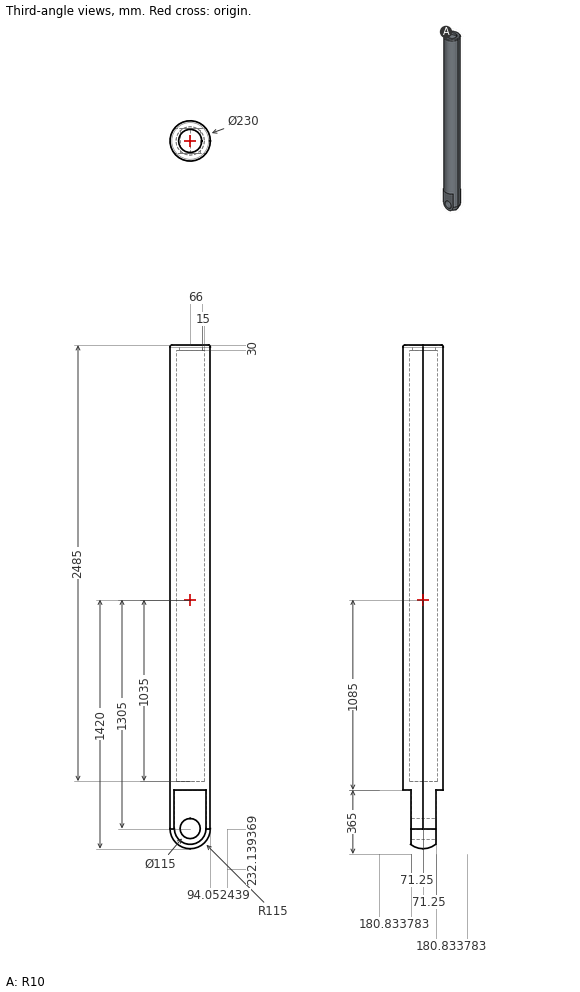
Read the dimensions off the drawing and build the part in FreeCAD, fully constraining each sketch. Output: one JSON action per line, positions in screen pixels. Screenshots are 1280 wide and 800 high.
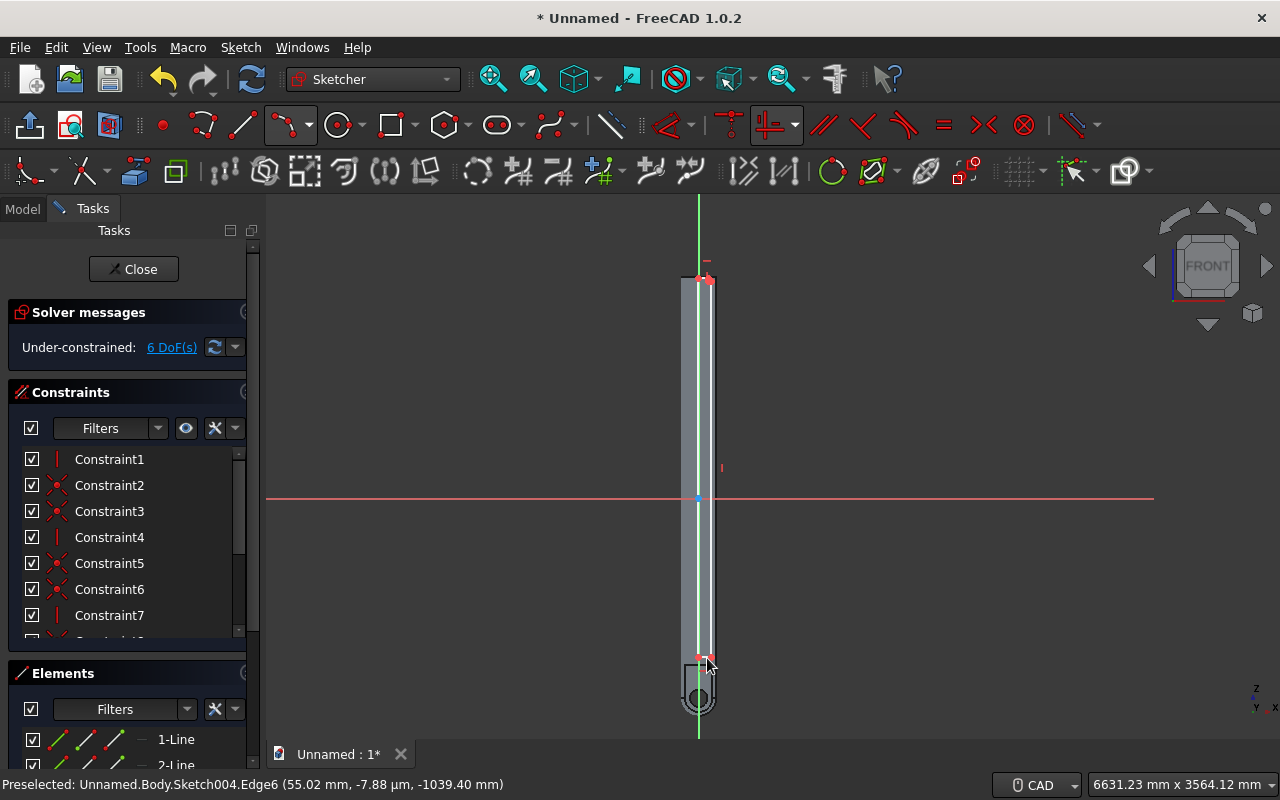
{"action": "left_click", "coordinate": [698, 657]}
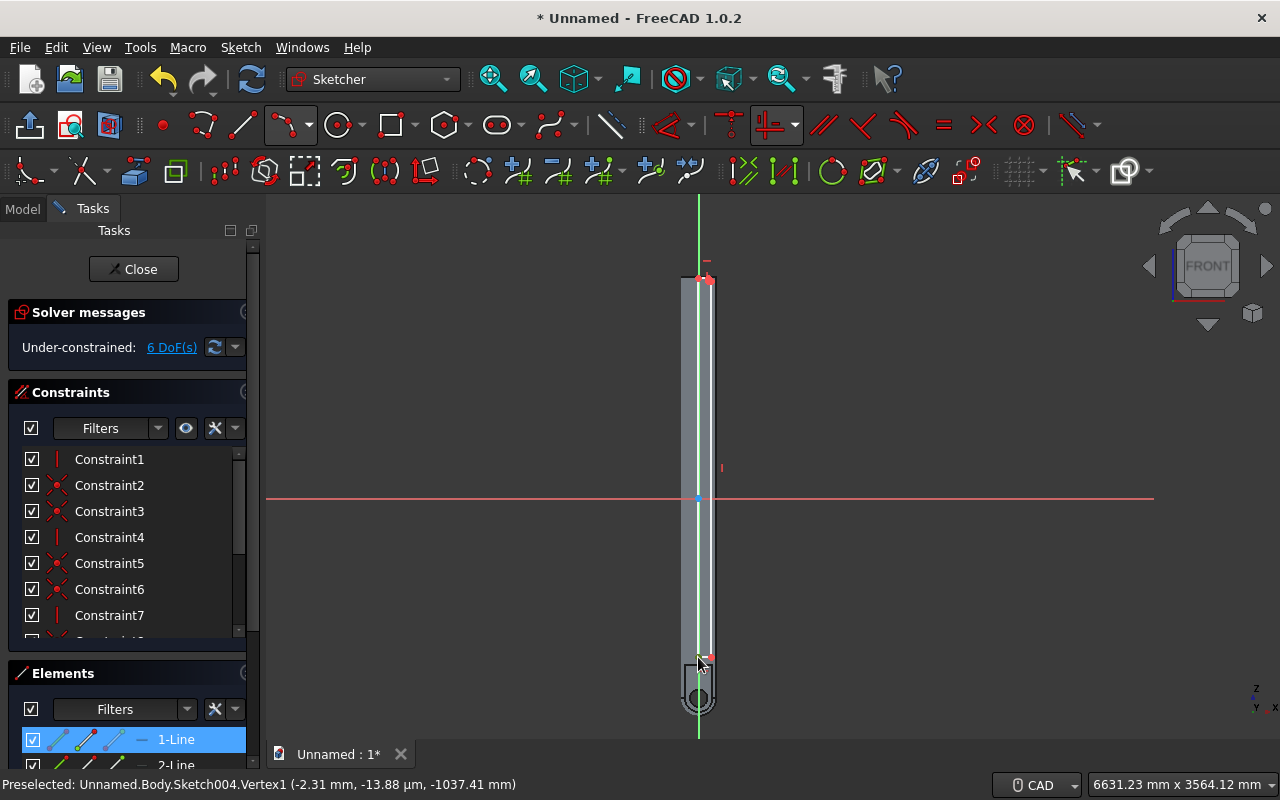
{"action": "left_click", "coordinate": [699, 257]}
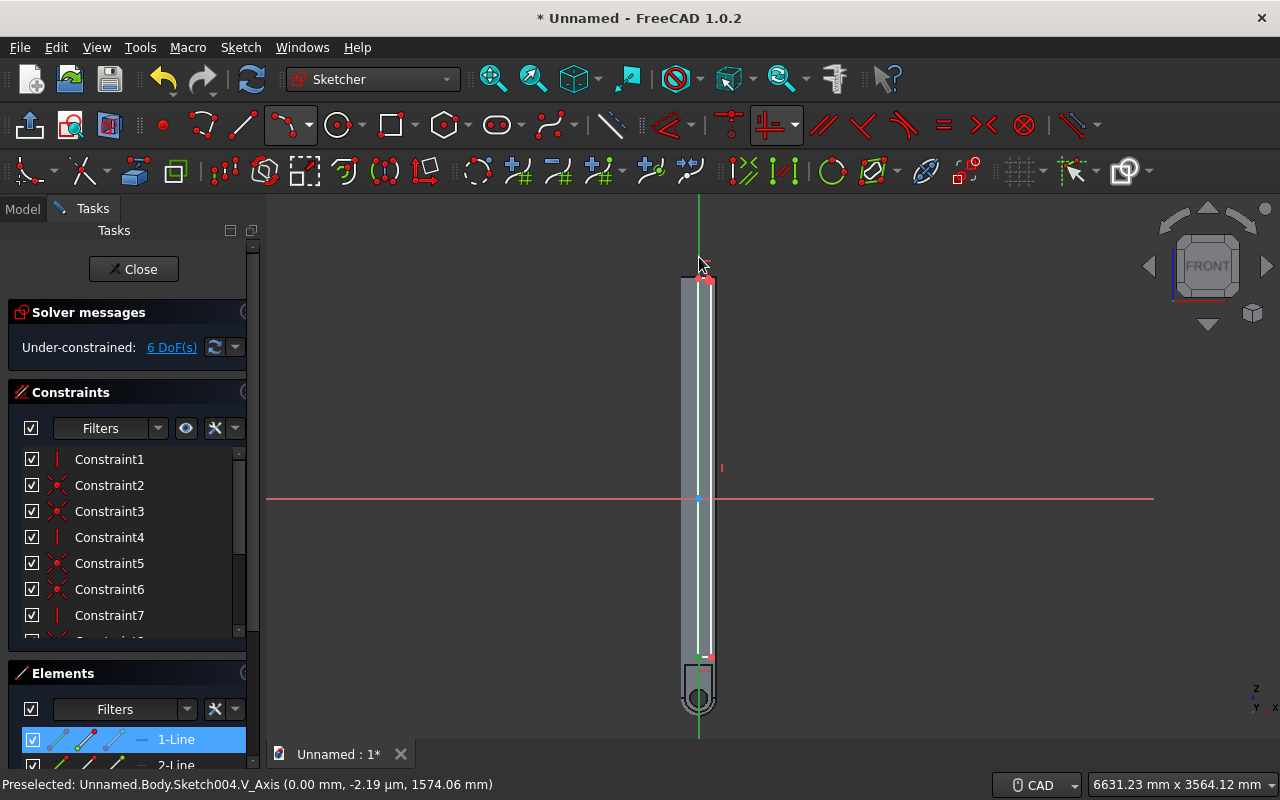
{"action": "key", "text": "c"}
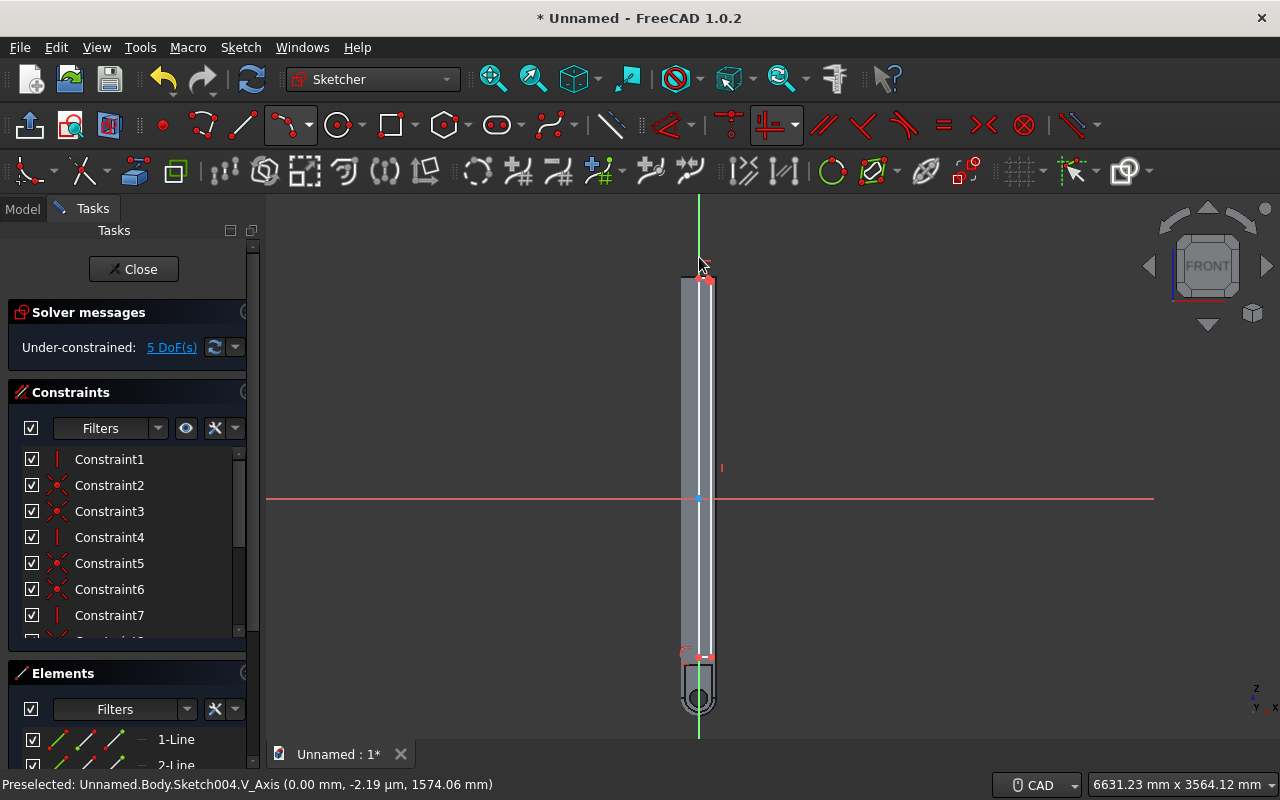
{"action": "key", "text": "d"}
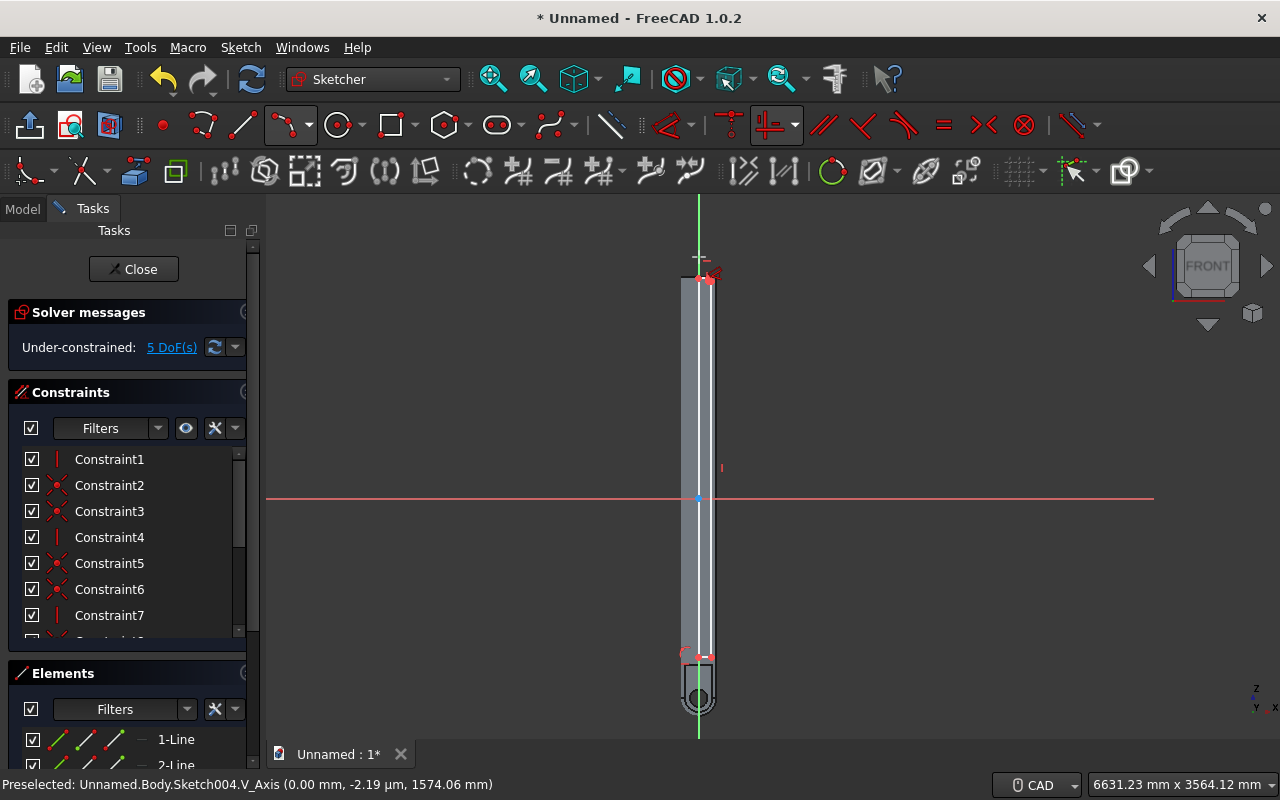
{"action": "scroll", "coordinate": [704, 278], "scroll_direction": "up", "scroll_amount": 7}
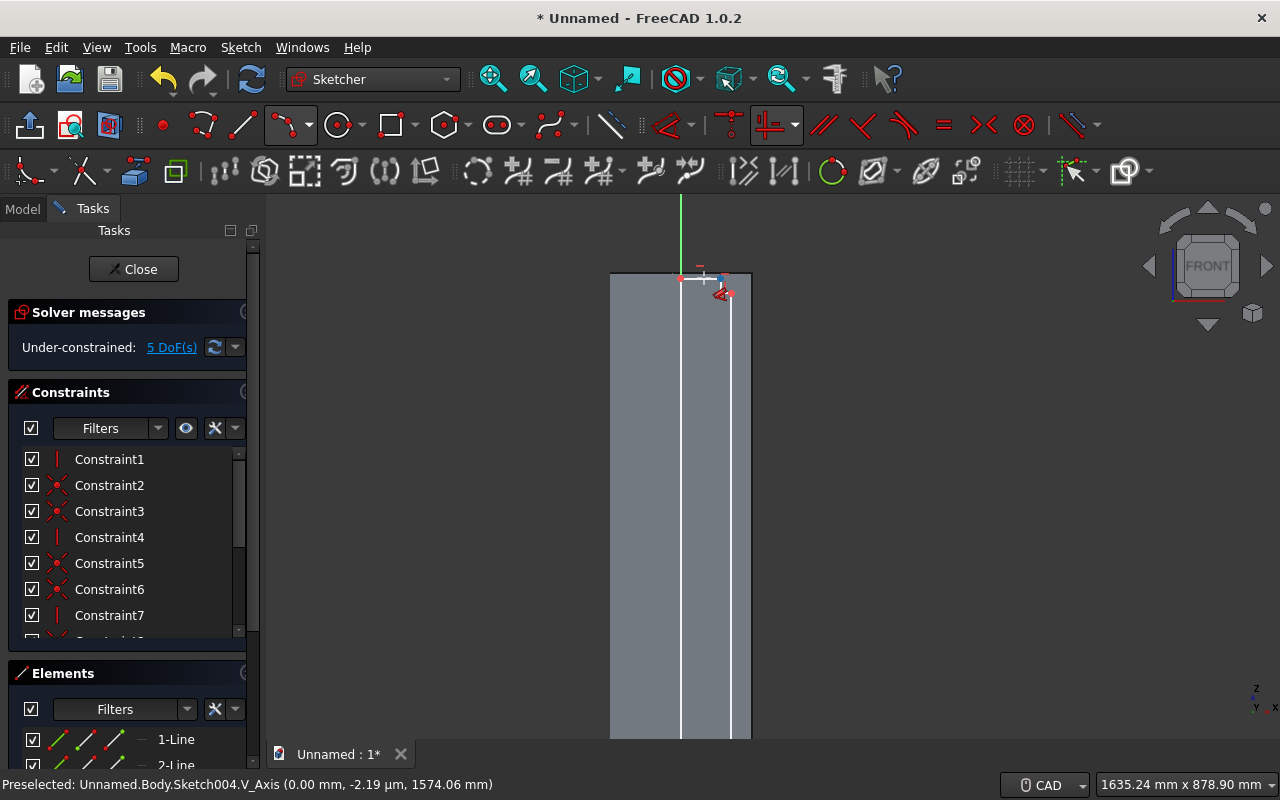
{"action": "left_click", "coordinate": [701, 279]}
{"action": "left_click", "coordinate": [701, 245]}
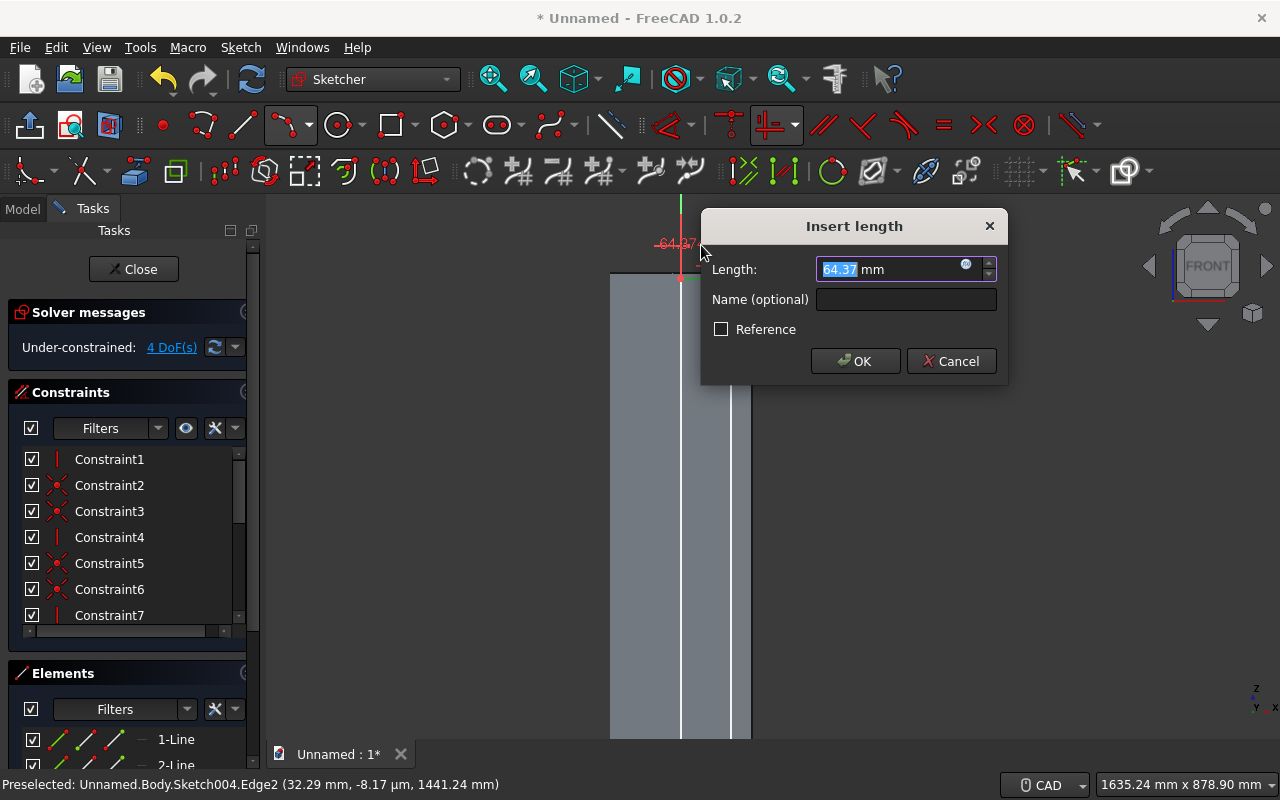
{"action": "type", "text": "66"}
{"action": "key", "text": "Return"}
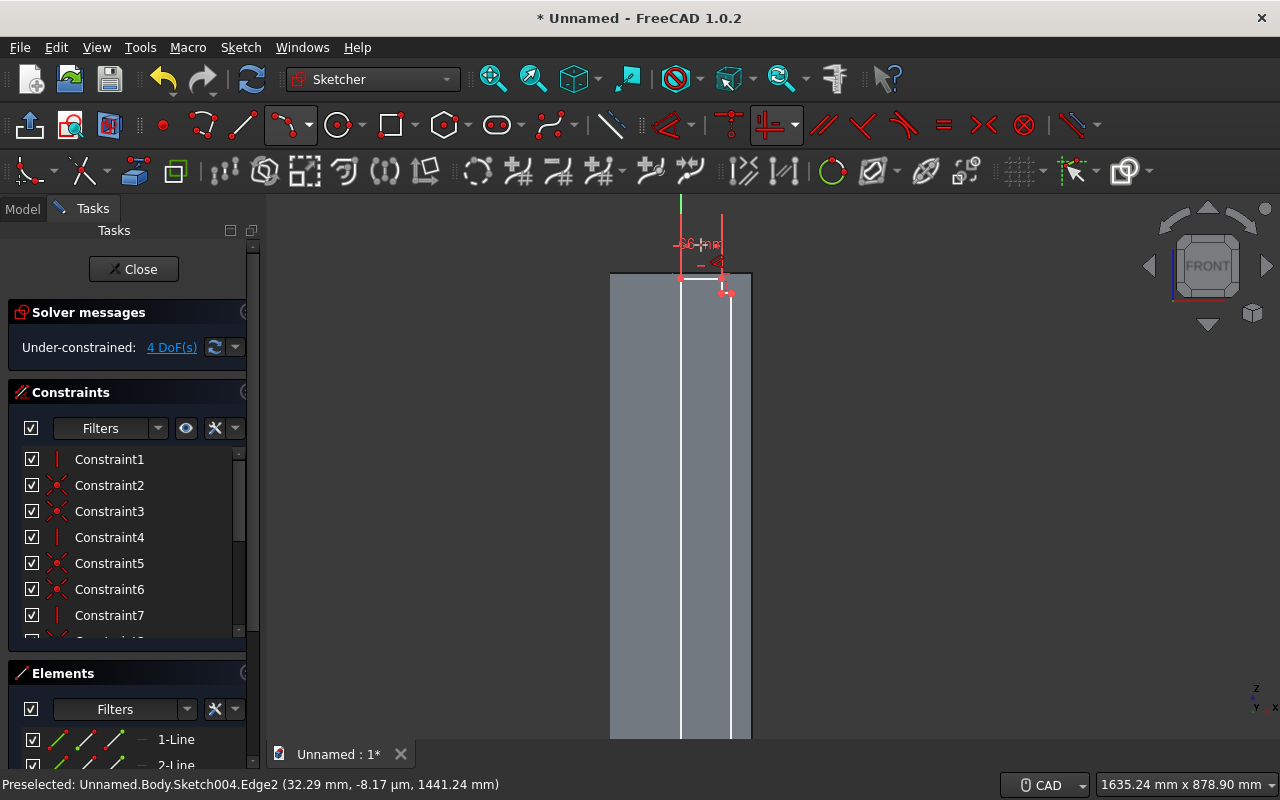
{"action": "scroll", "coordinate": [722, 286], "scroll_direction": "up", "scroll_amount": 4}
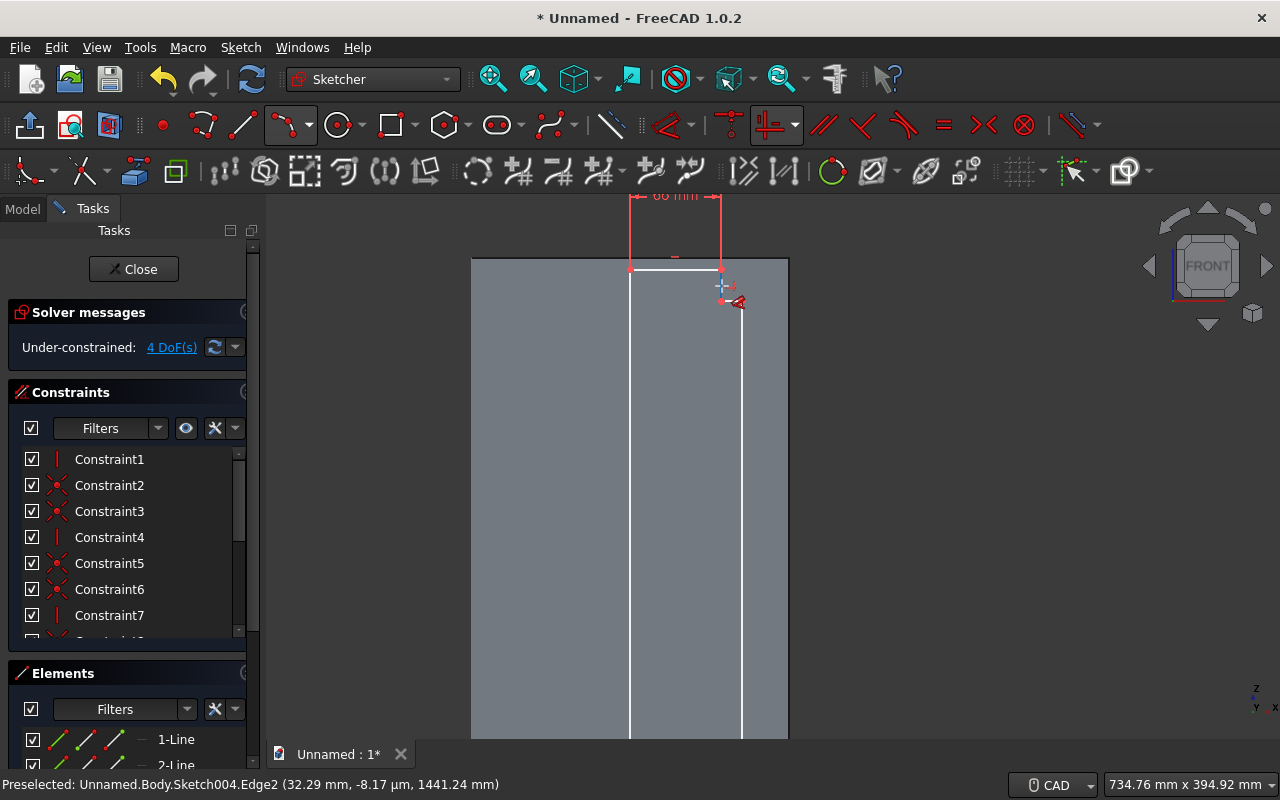
{"action": "left_click", "coordinate": [721, 286]}
{"action": "left_click", "coordinate": [755, 286]}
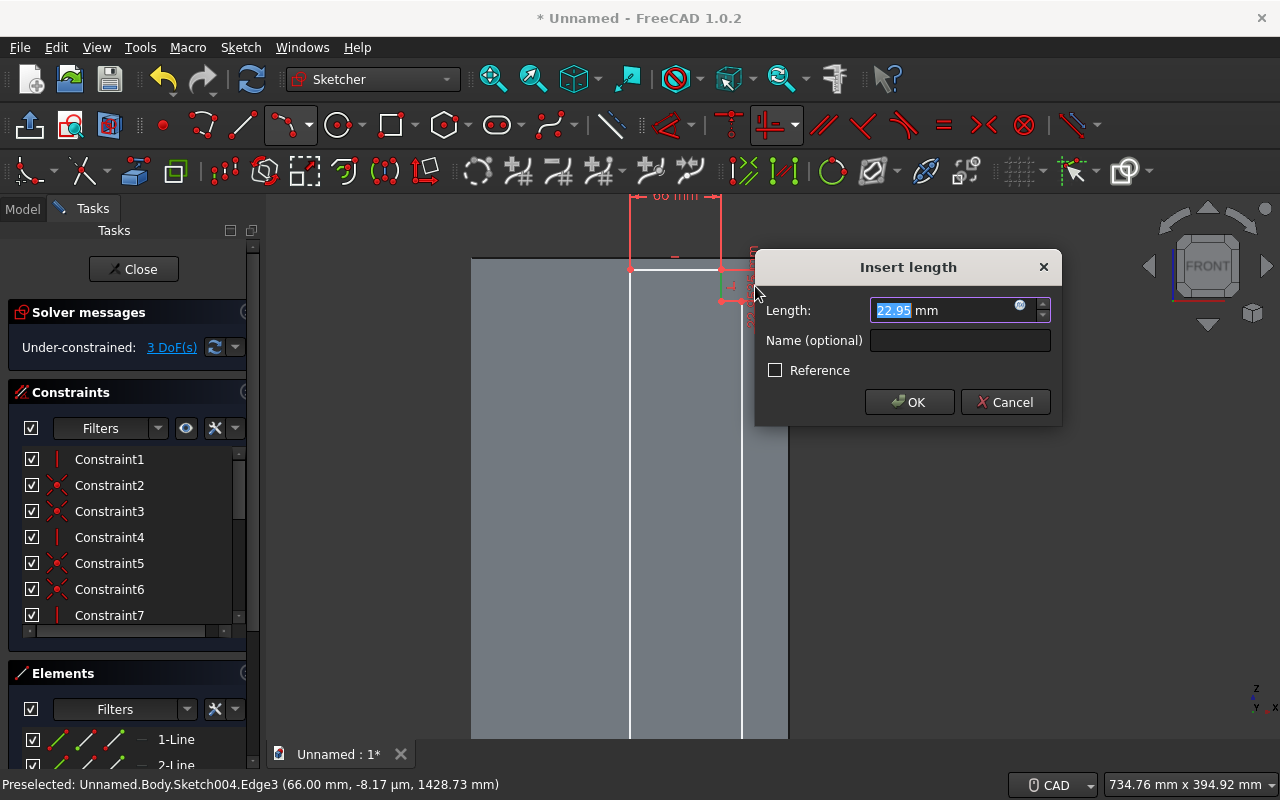
{"action": "type", "text": "30"}
{"action": "key", "text": "Return"}